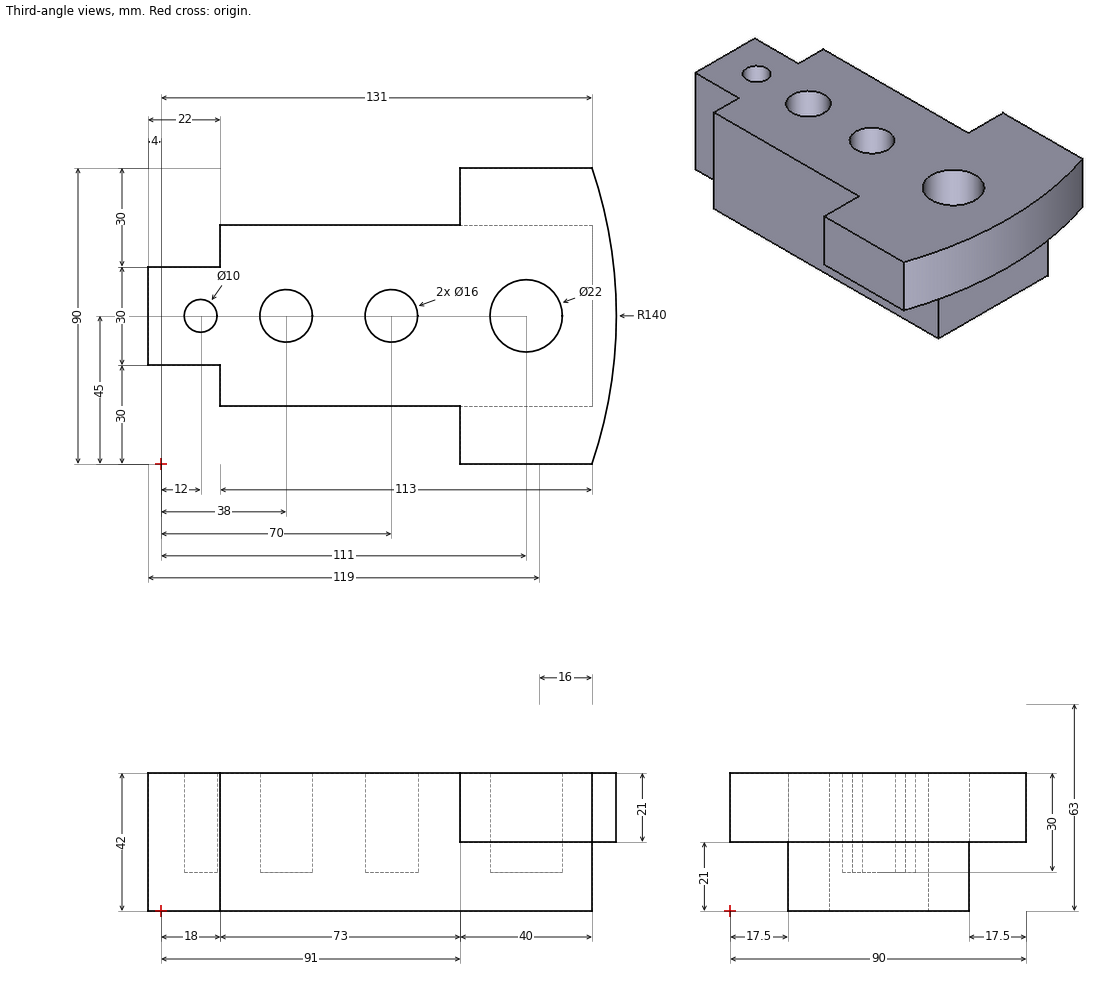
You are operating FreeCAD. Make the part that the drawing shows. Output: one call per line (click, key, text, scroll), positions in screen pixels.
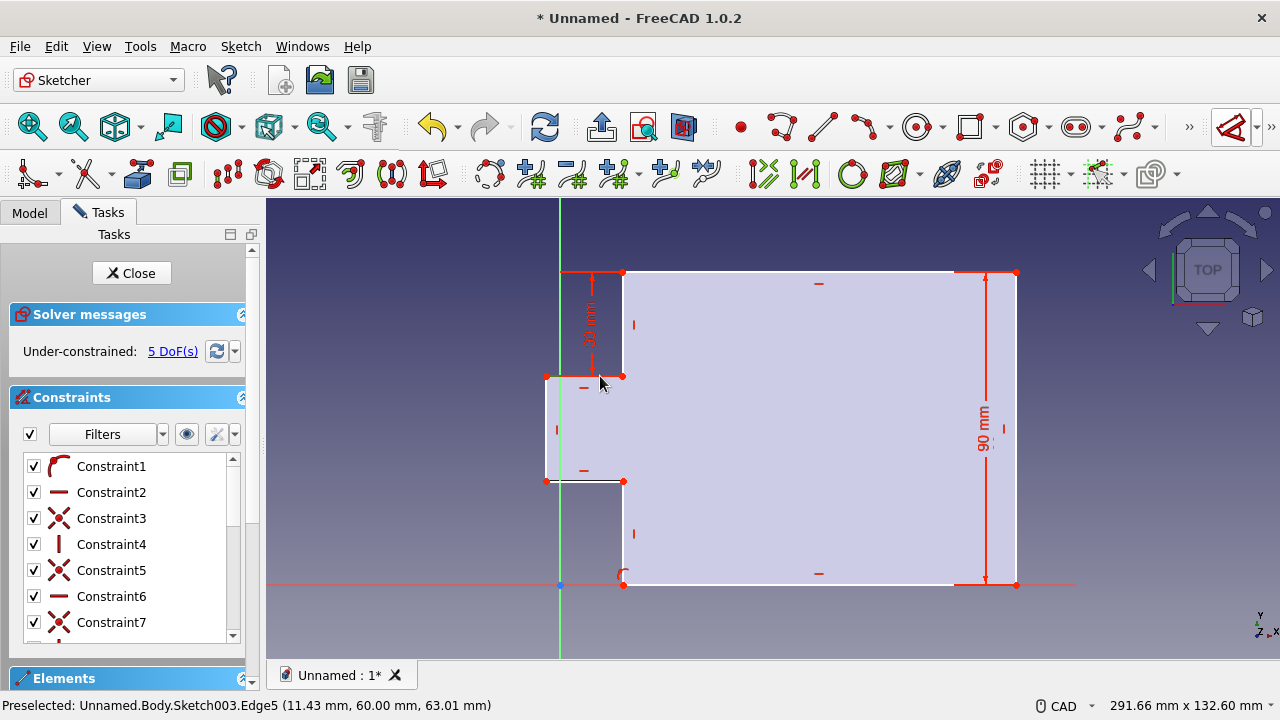
key(l)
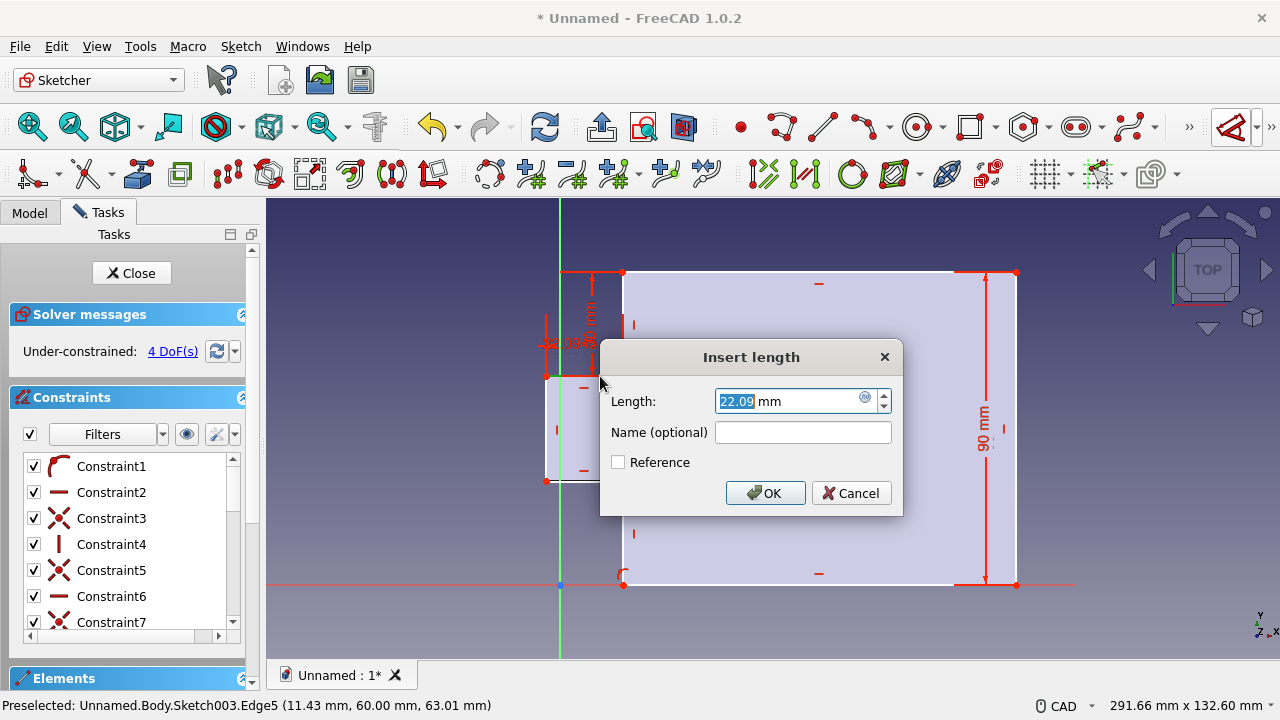
text(22)
key(Return)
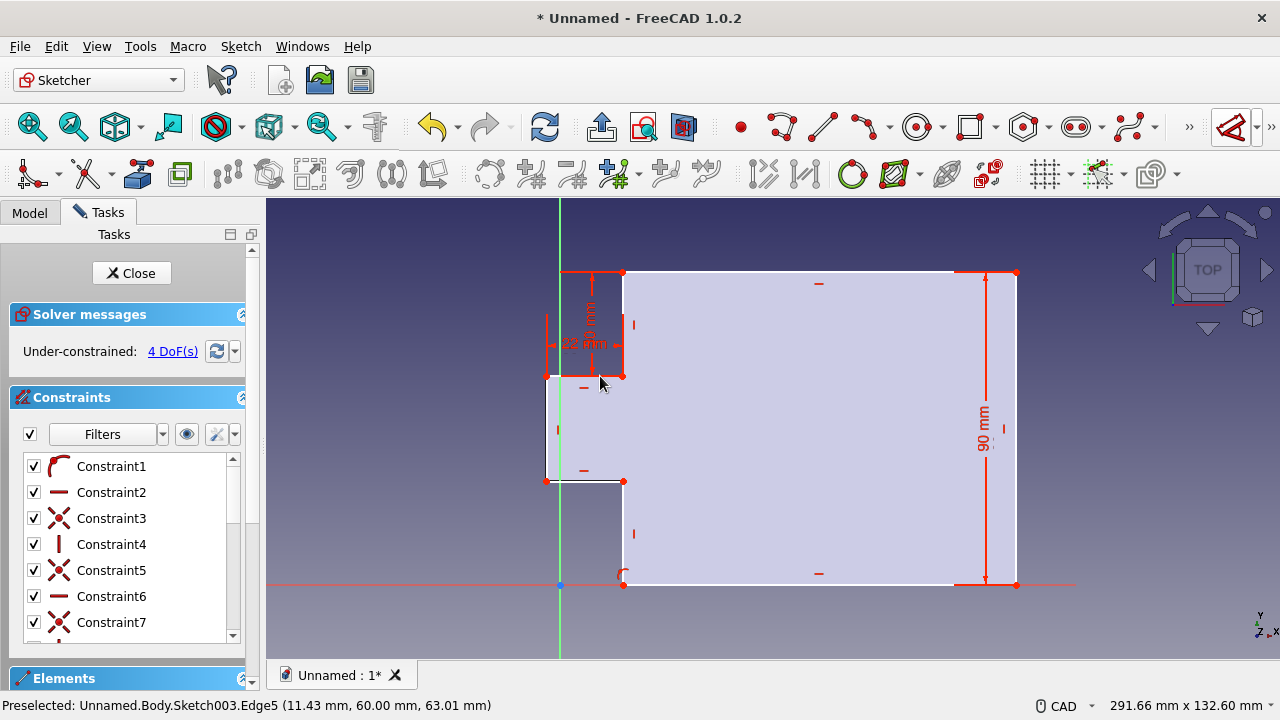
click(547, 408)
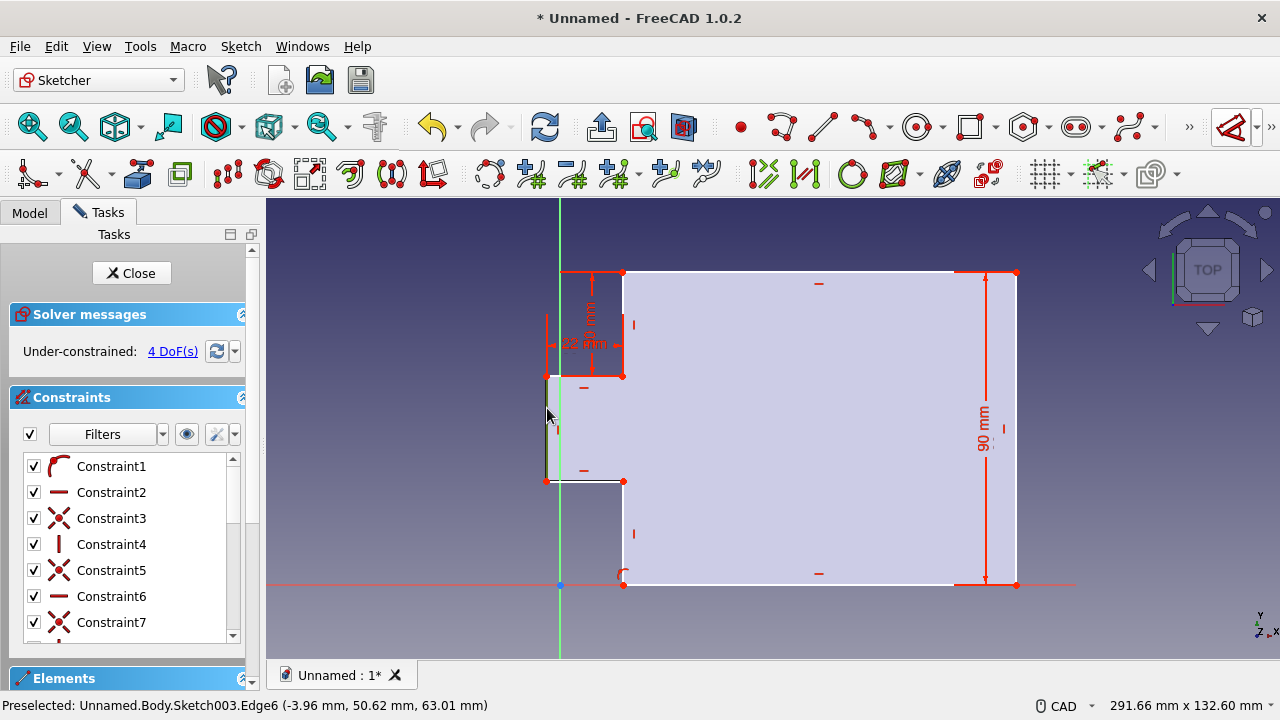
click(1256, 128)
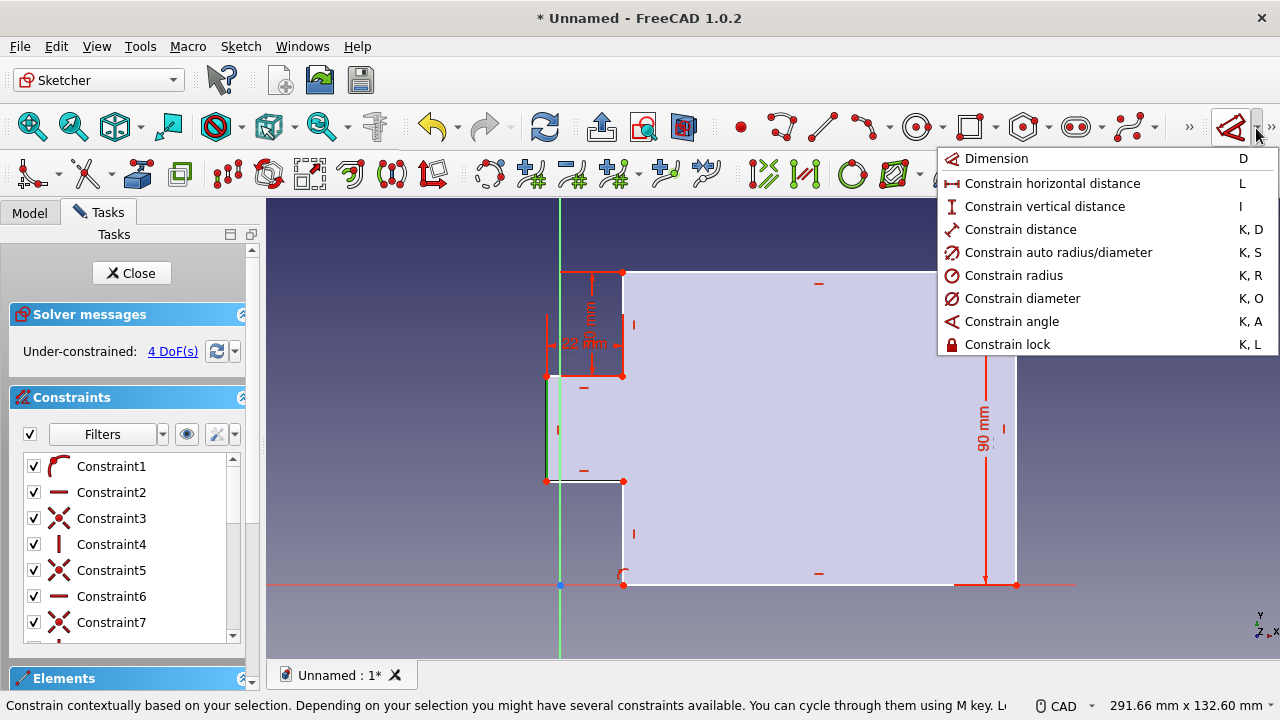
click(1108, 206)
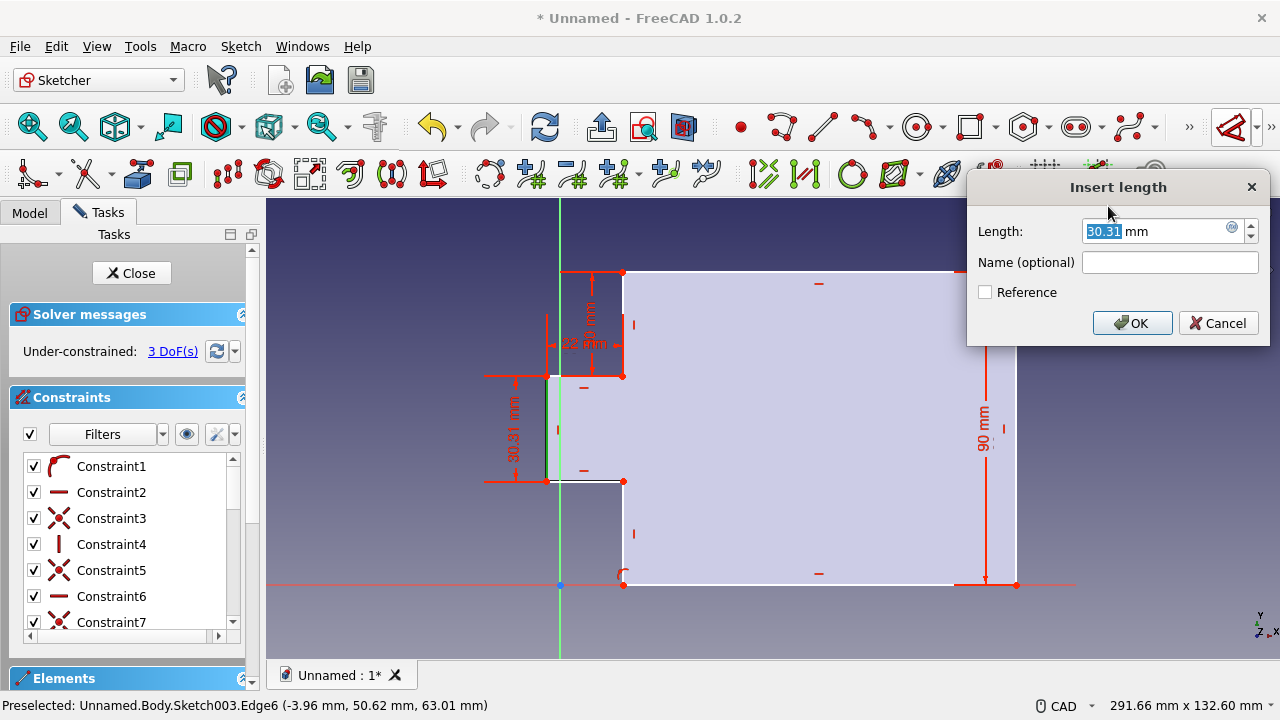
text(30)
key(Return)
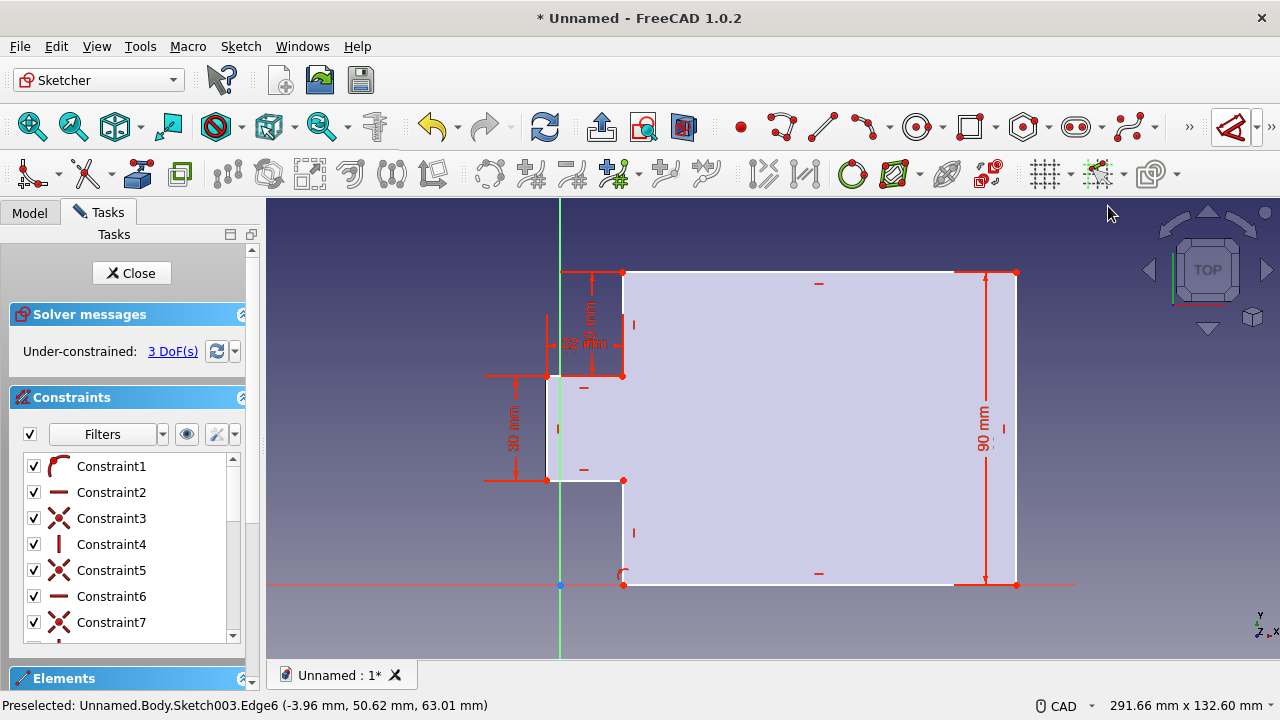
scroll(569, 481, up, 3)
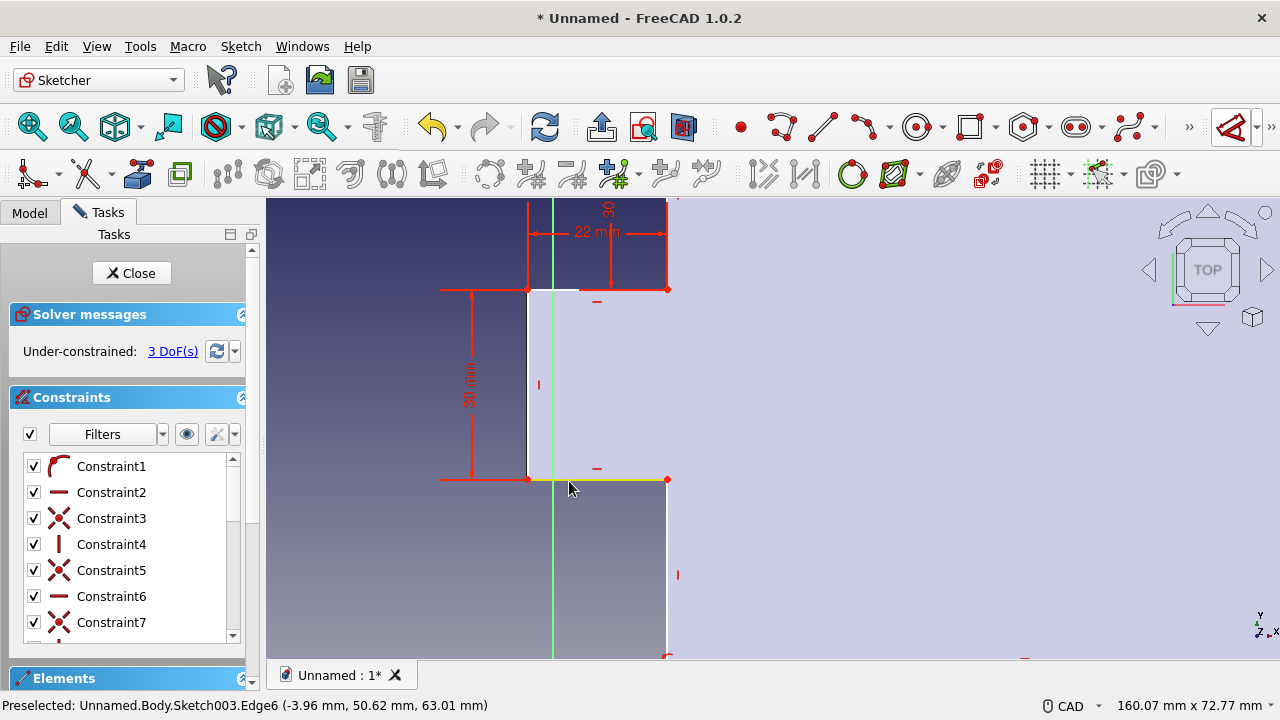
click(570, 480)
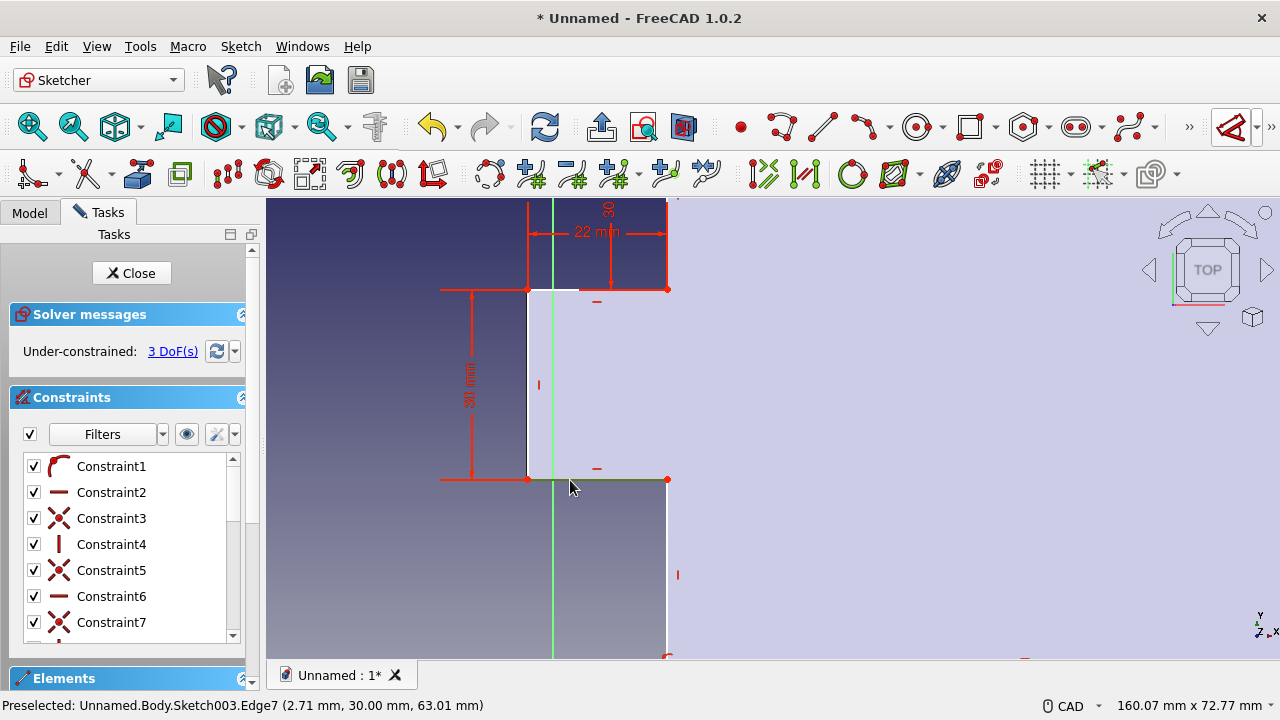
click(1256, 128)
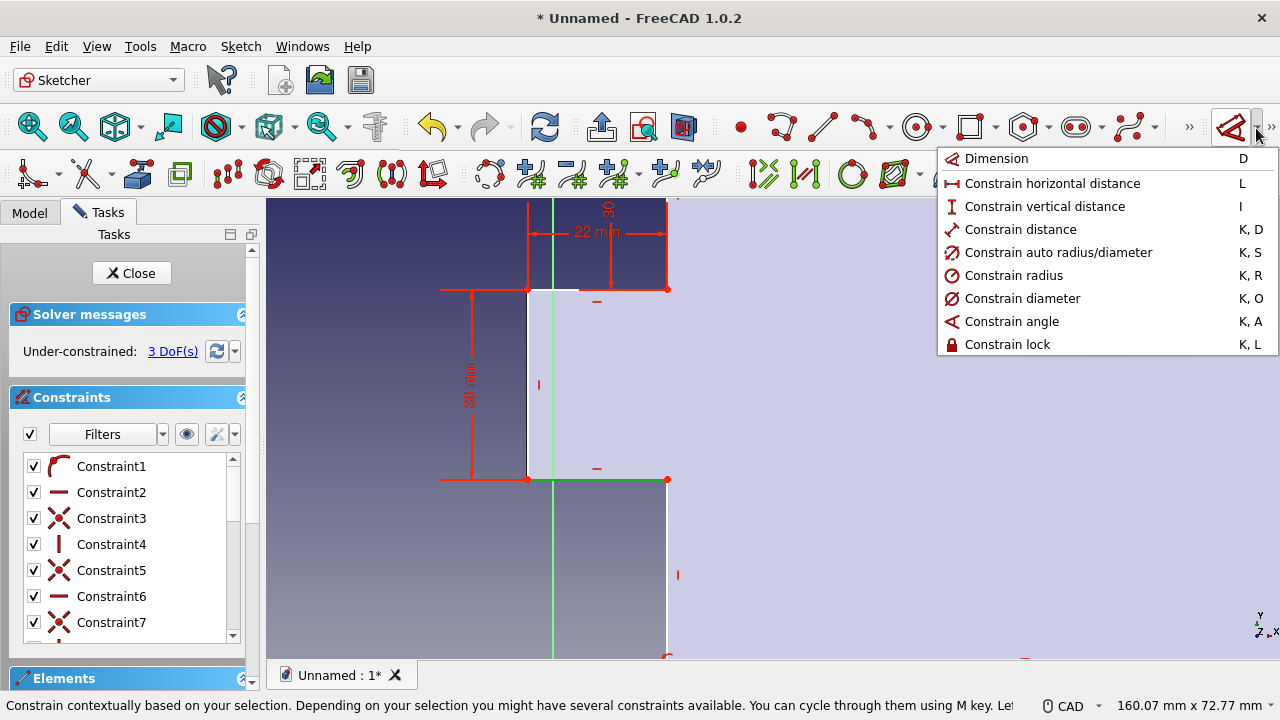
click(1108, 184)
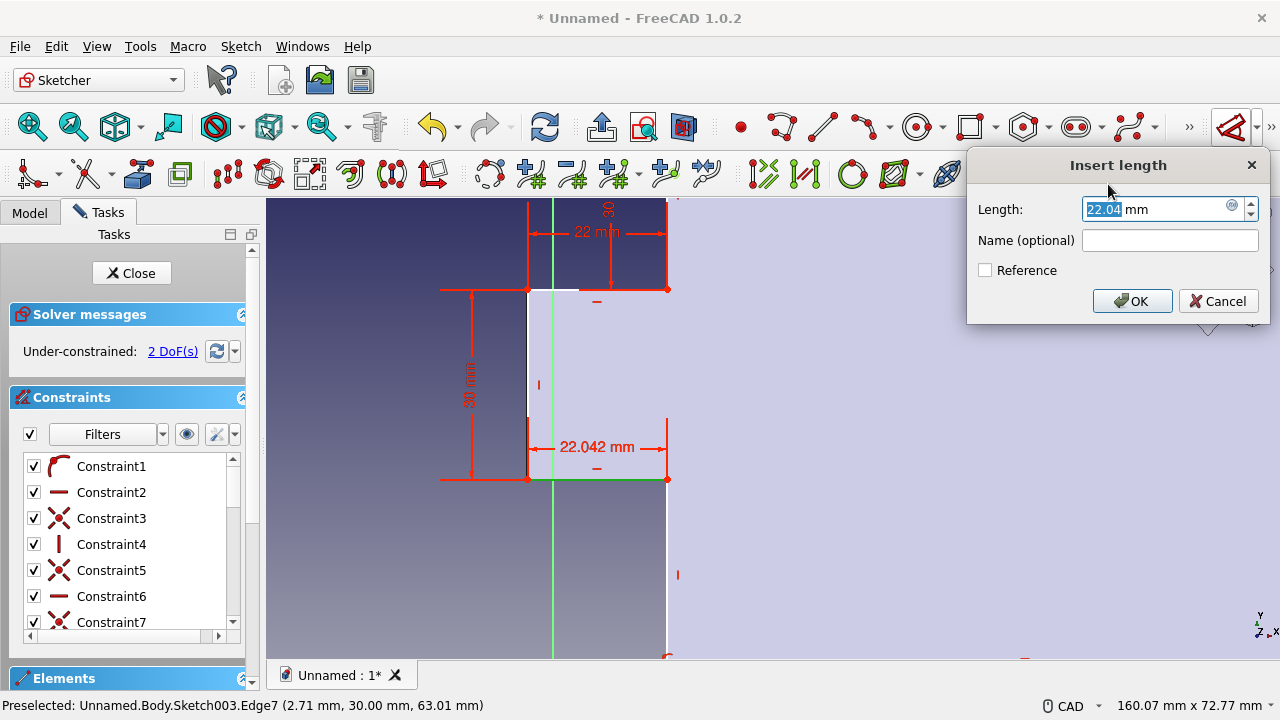
text(22)
key(Return)